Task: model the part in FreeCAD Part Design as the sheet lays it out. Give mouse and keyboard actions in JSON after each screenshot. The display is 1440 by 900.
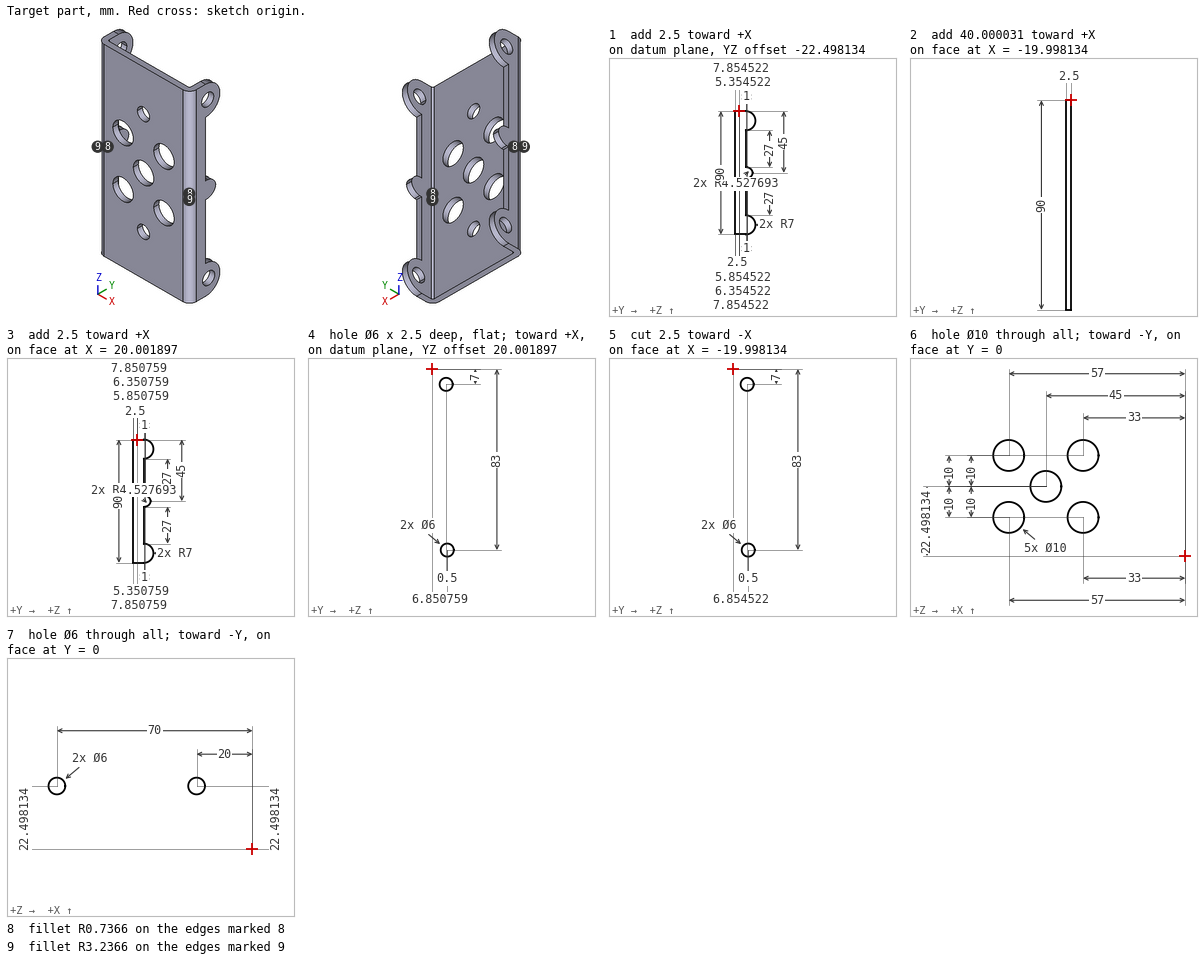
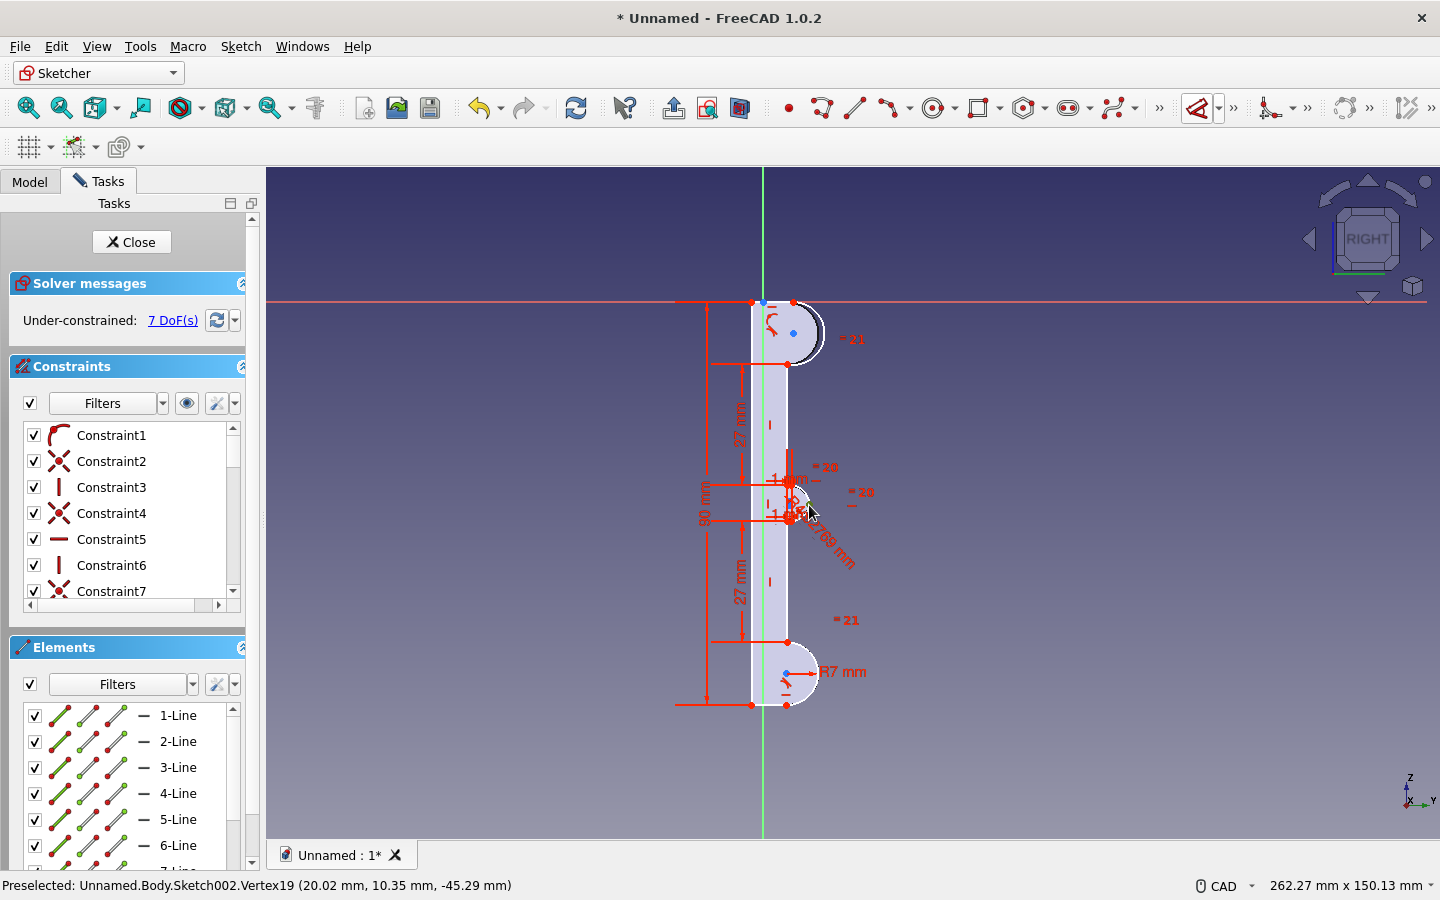
{"action": "left_click", "coordinate": [1218, 108]}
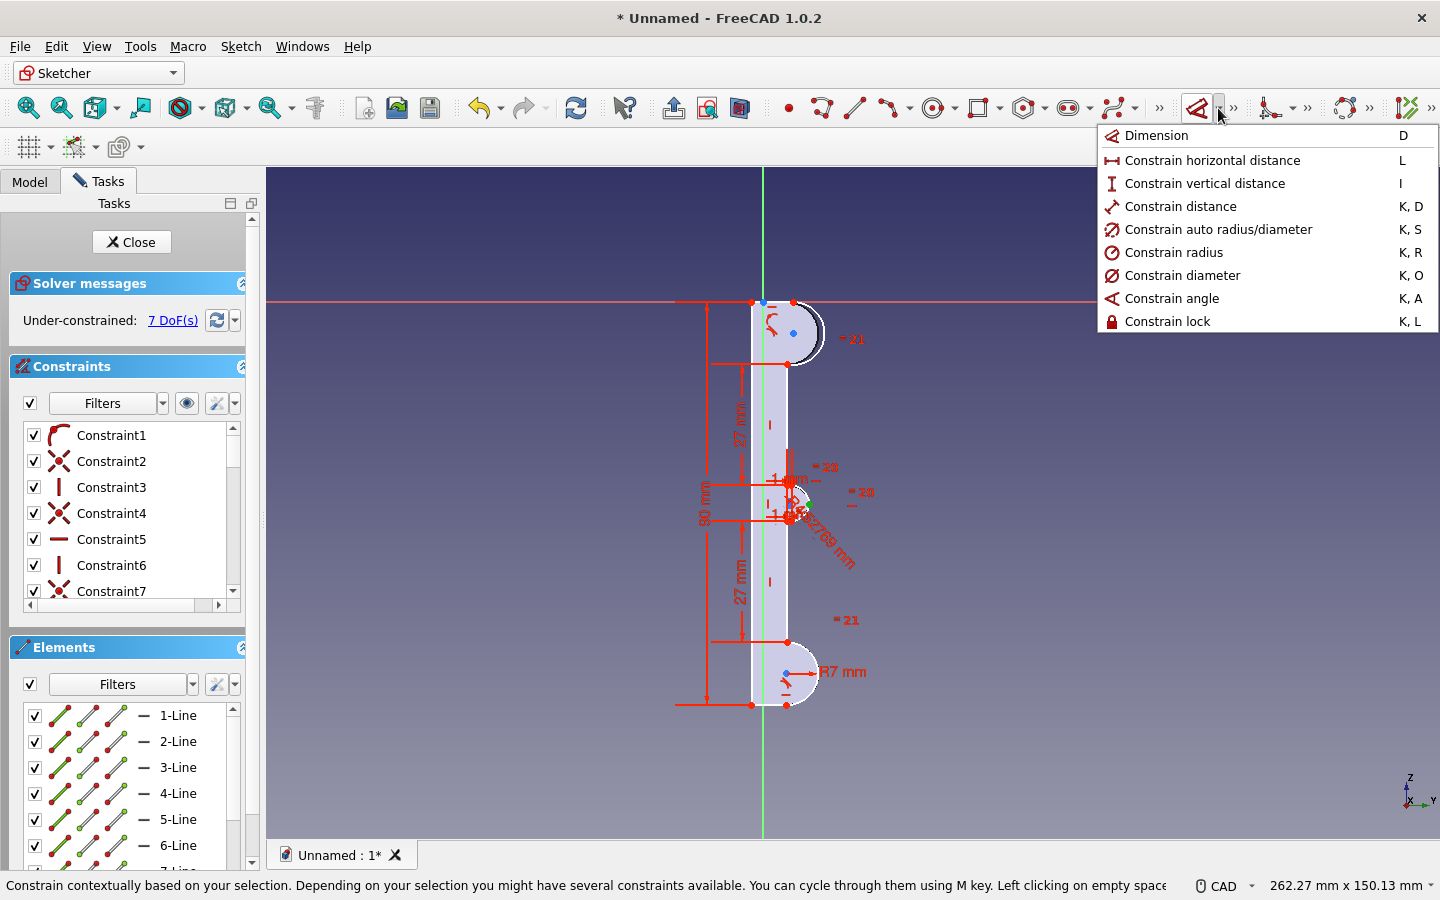
{"action": "left_click", "coordinate": [1268, 184]}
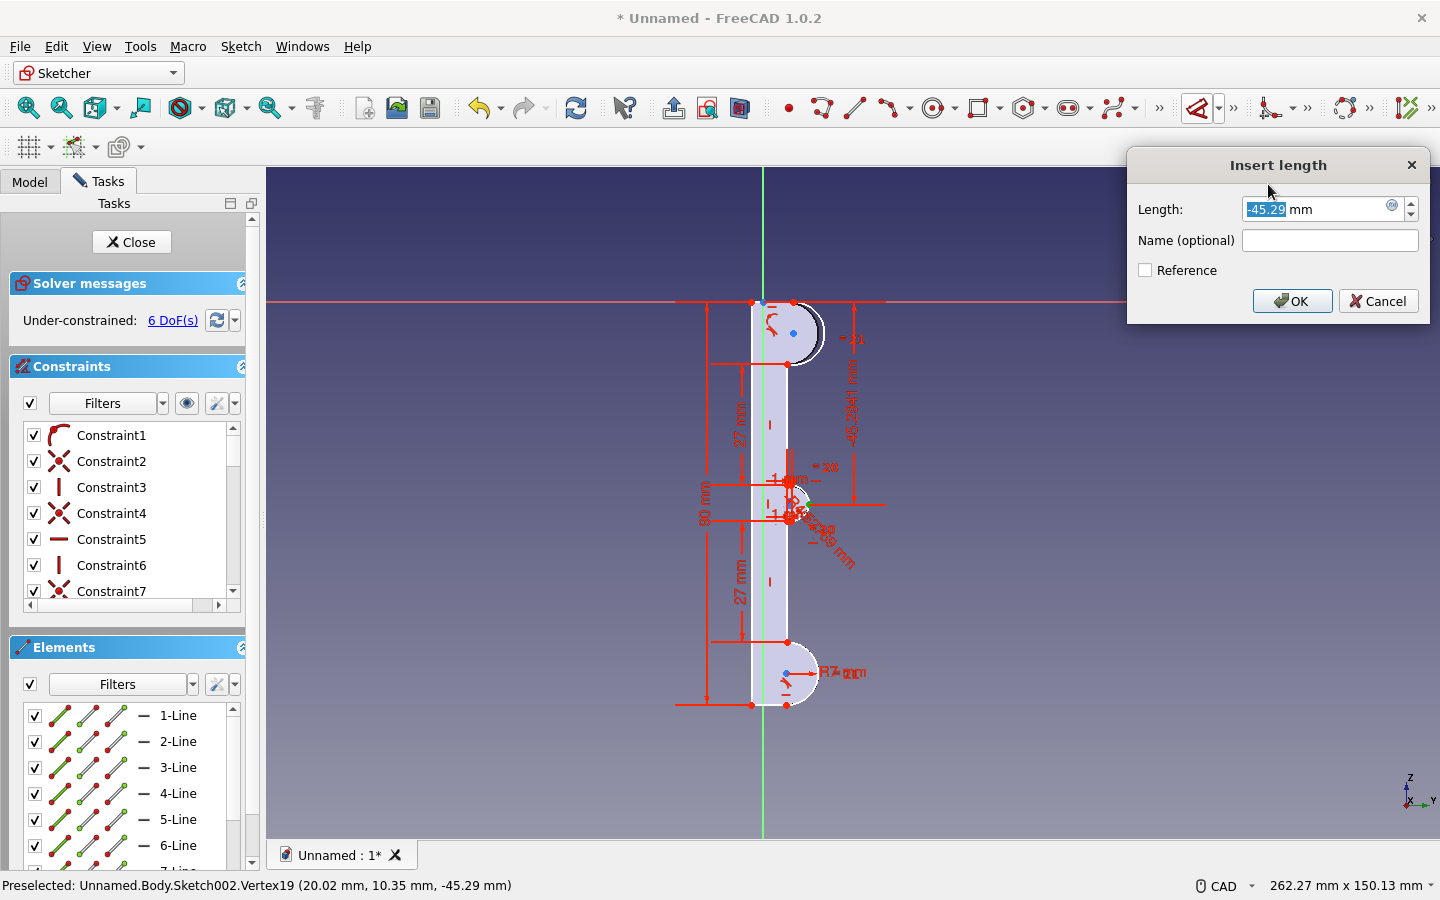
{"action": "type", "text": "-45"}
{"action": "key", "text": "Return"}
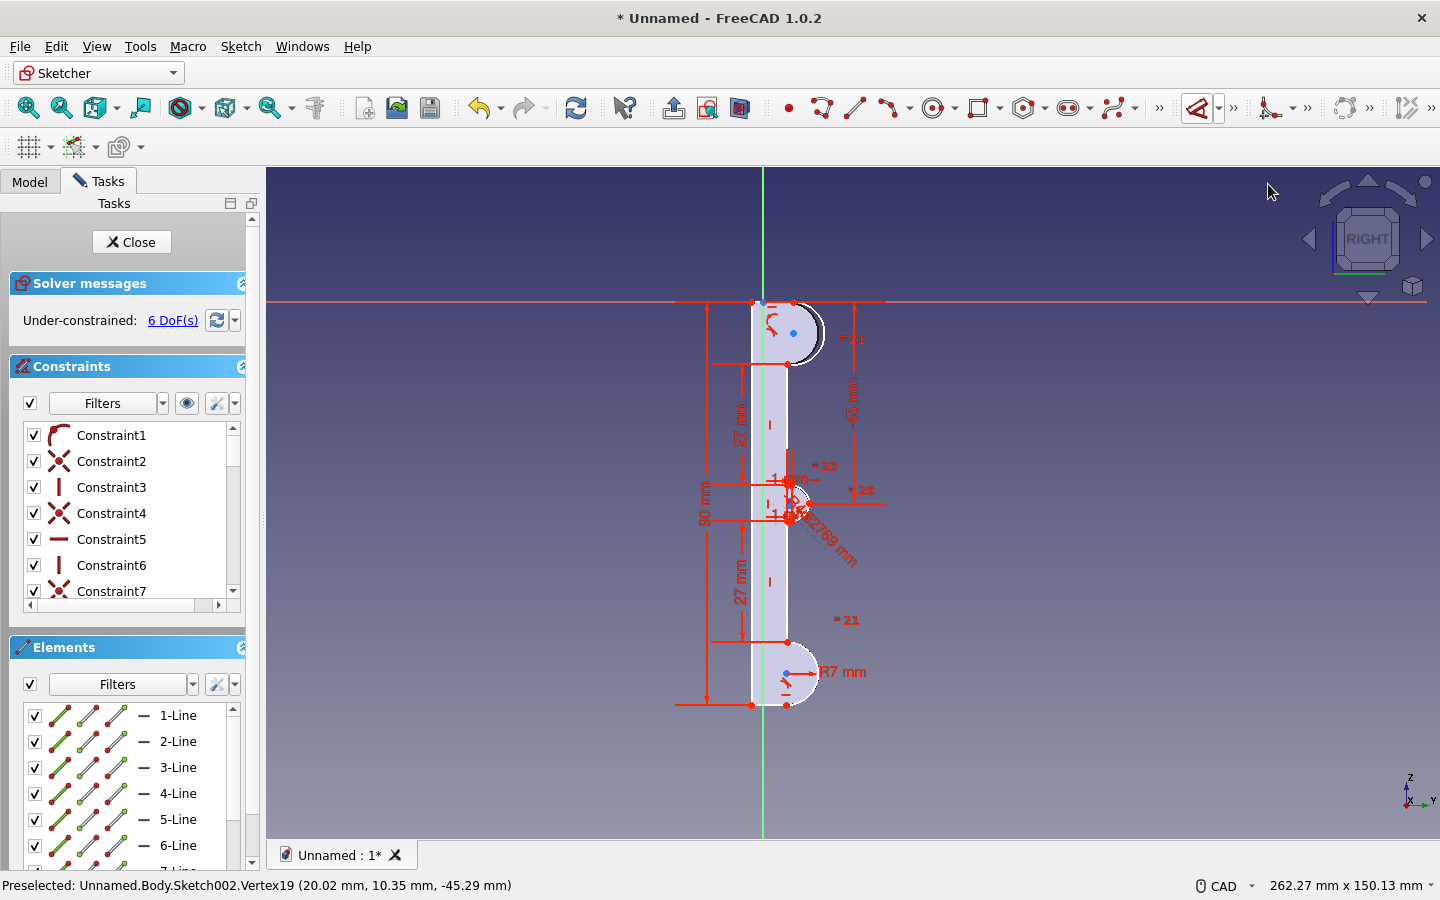
{"action": "scroll", "coordinate": [752, 302], "scroll_direction": "up", "scroll_amount": 7}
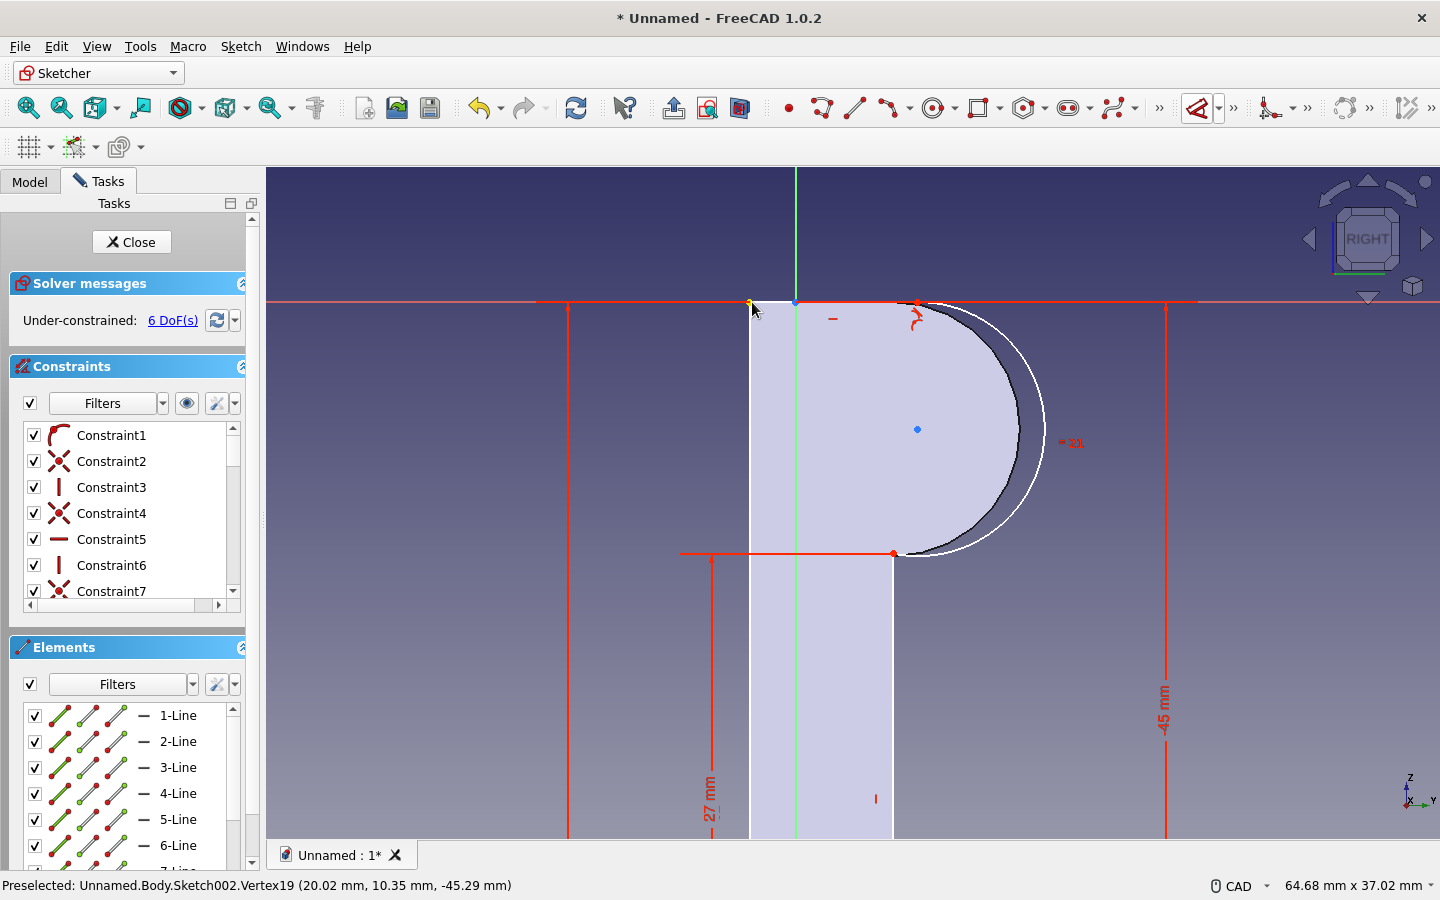
{"action": "left_click", "coordinate": [750, 302]}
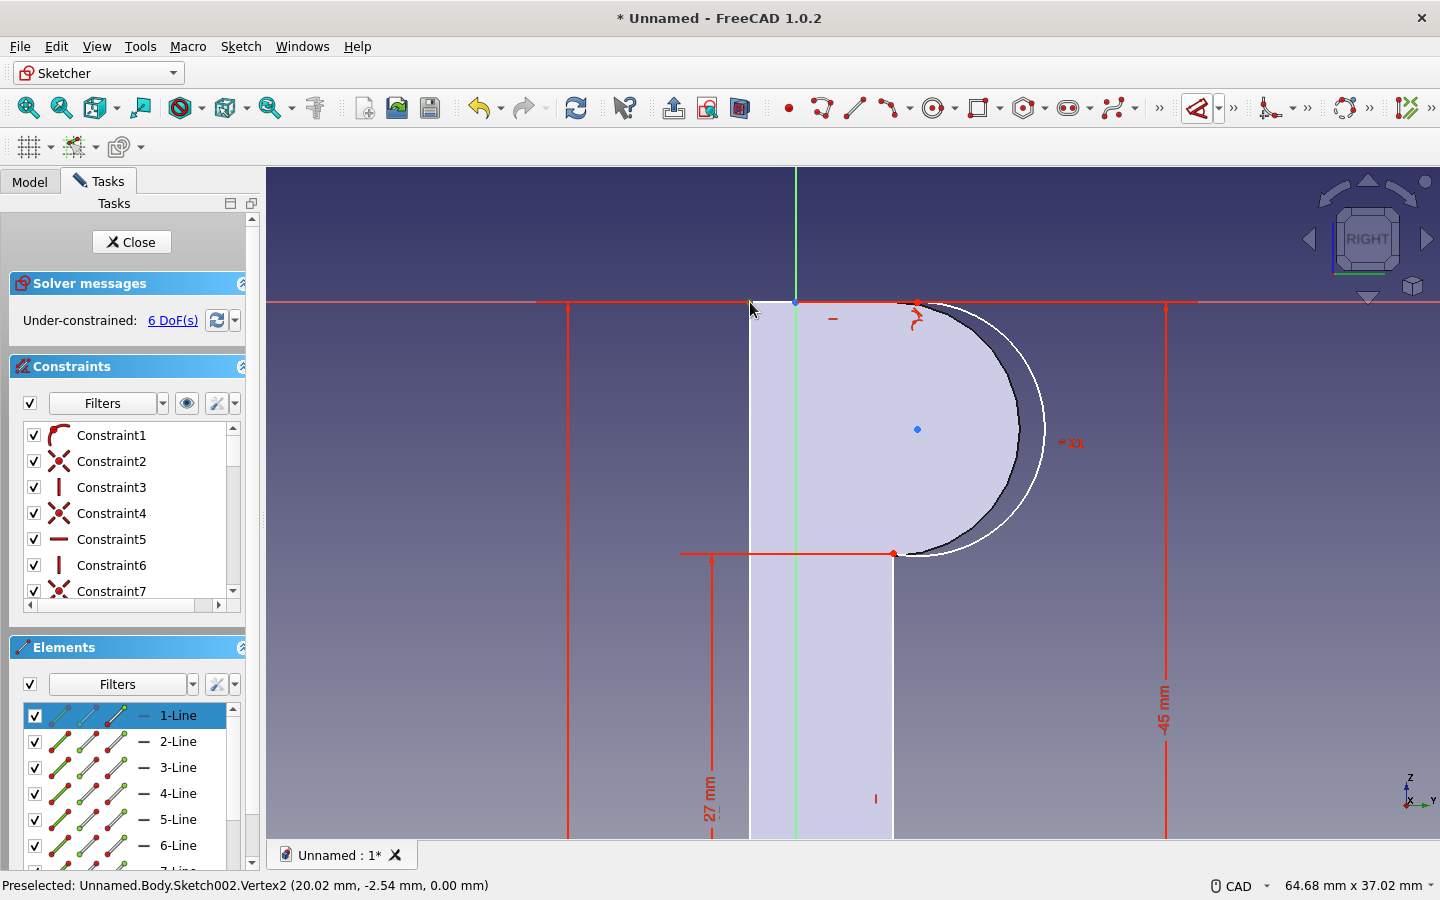
{"action": "key", "text": "l"}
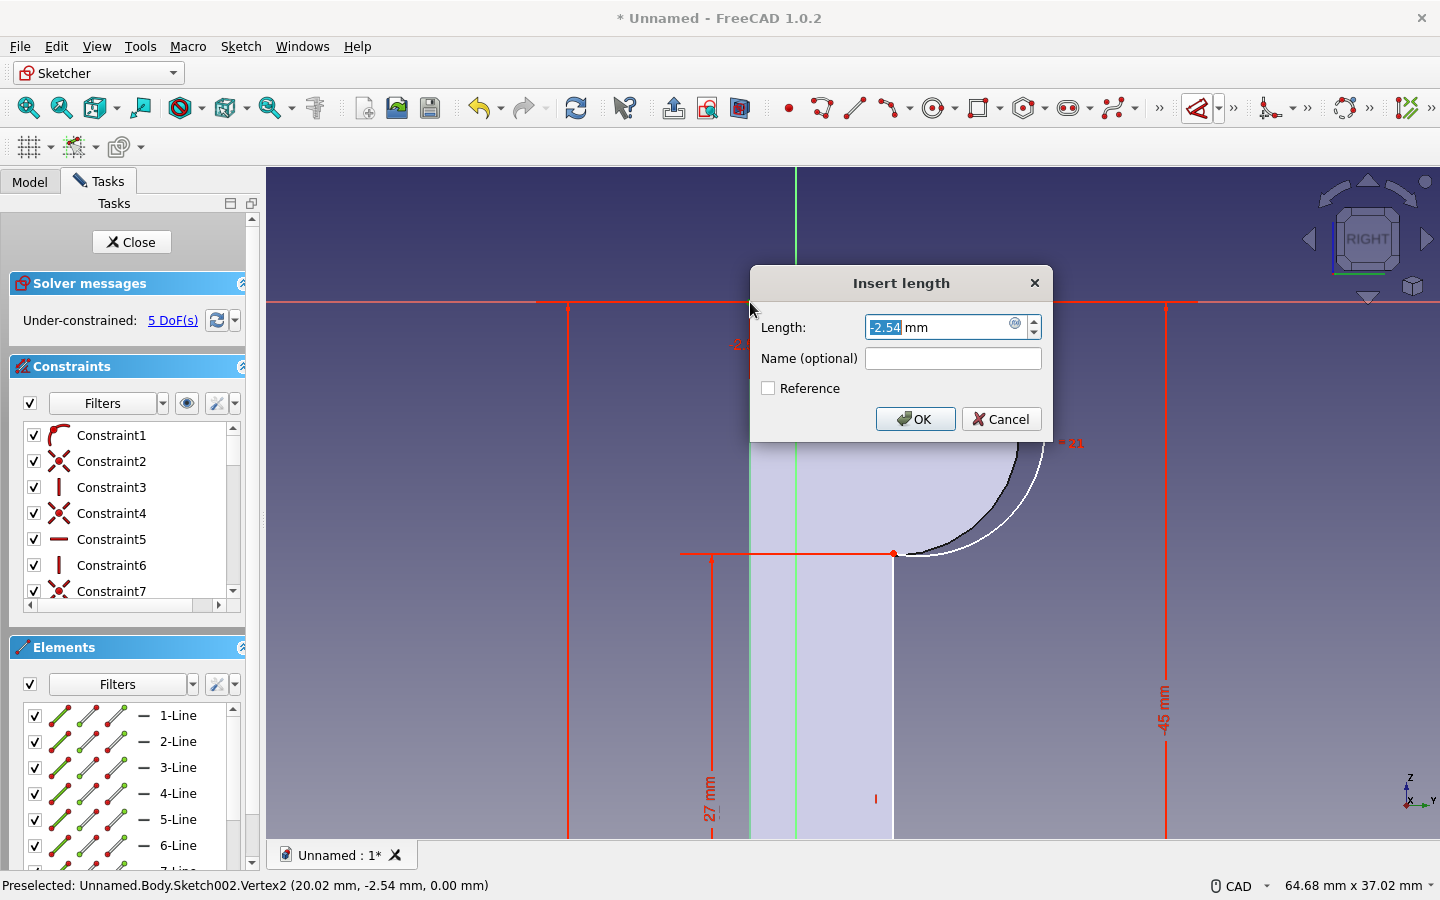
{"action": "type", "text": "-2.5"}
{"action": "key", "text": "Return"}